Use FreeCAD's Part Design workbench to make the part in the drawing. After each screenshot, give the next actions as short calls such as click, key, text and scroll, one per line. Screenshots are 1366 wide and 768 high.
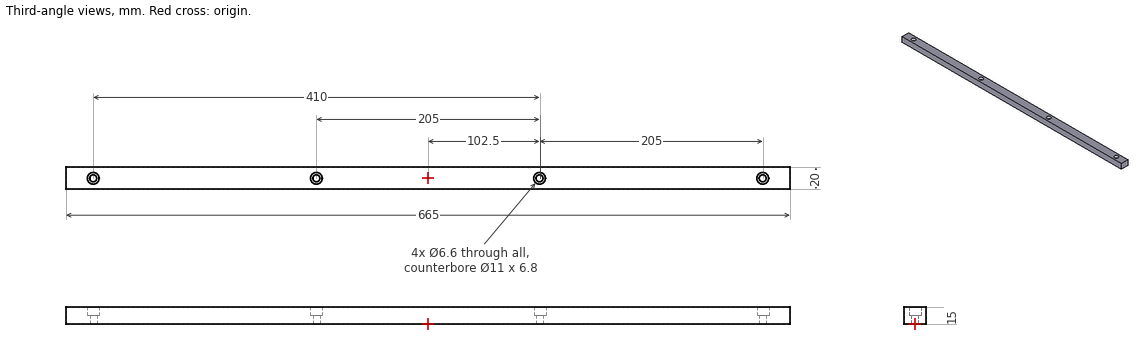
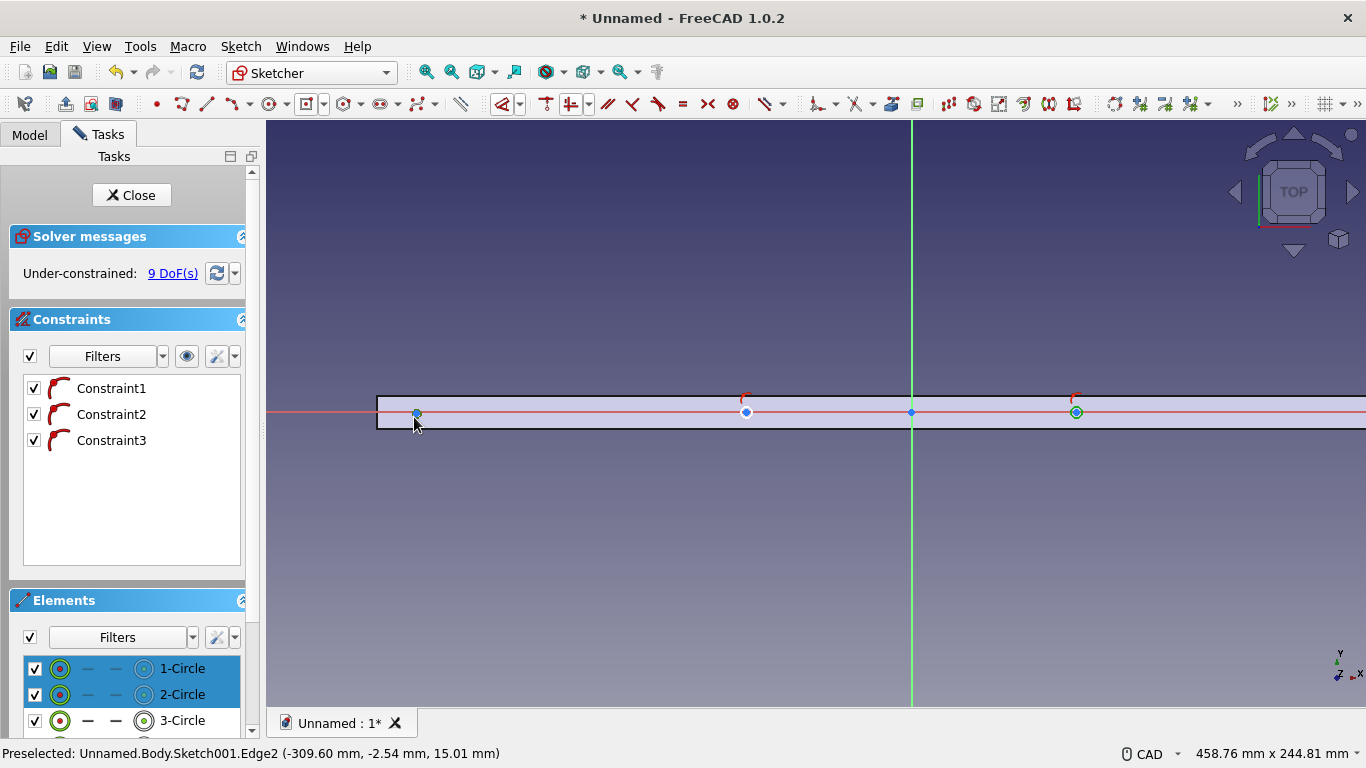
scroll(1082, 411, up, 9)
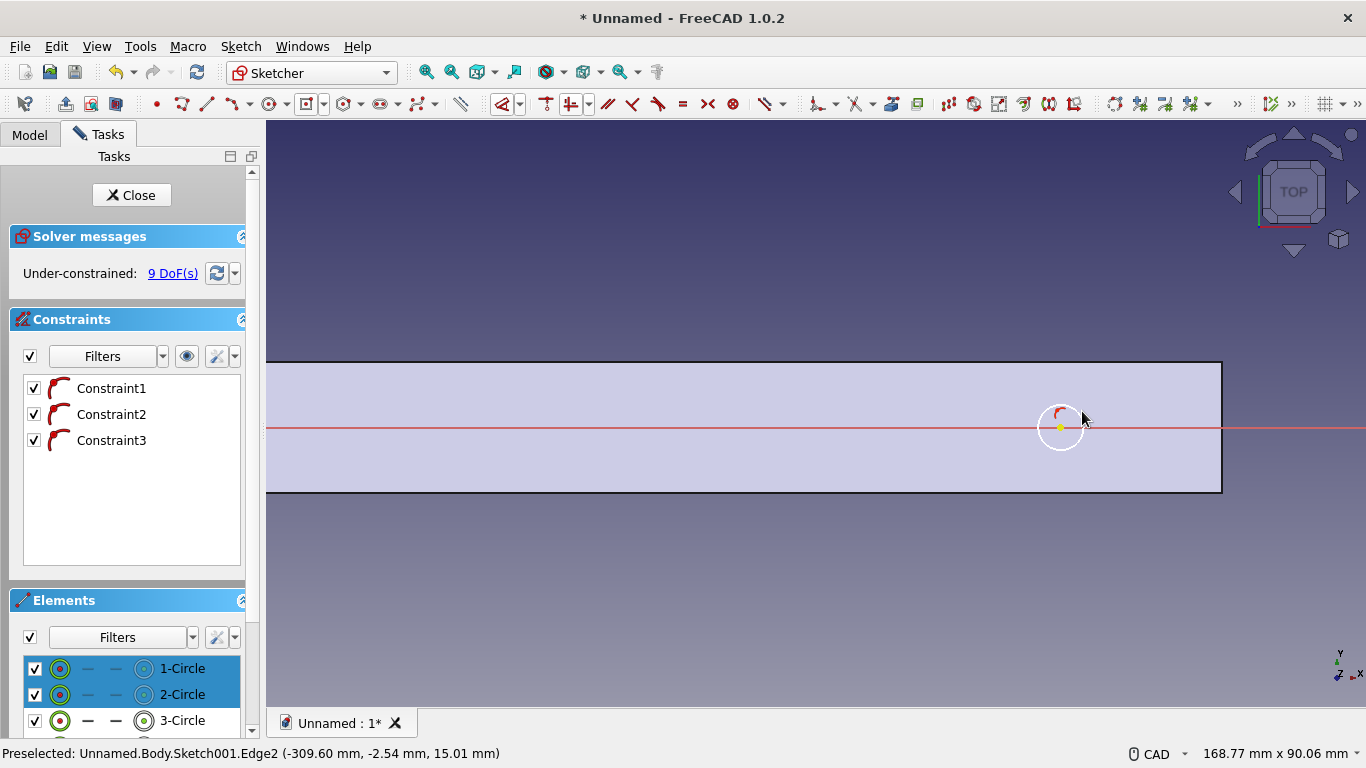
click(1077, 411)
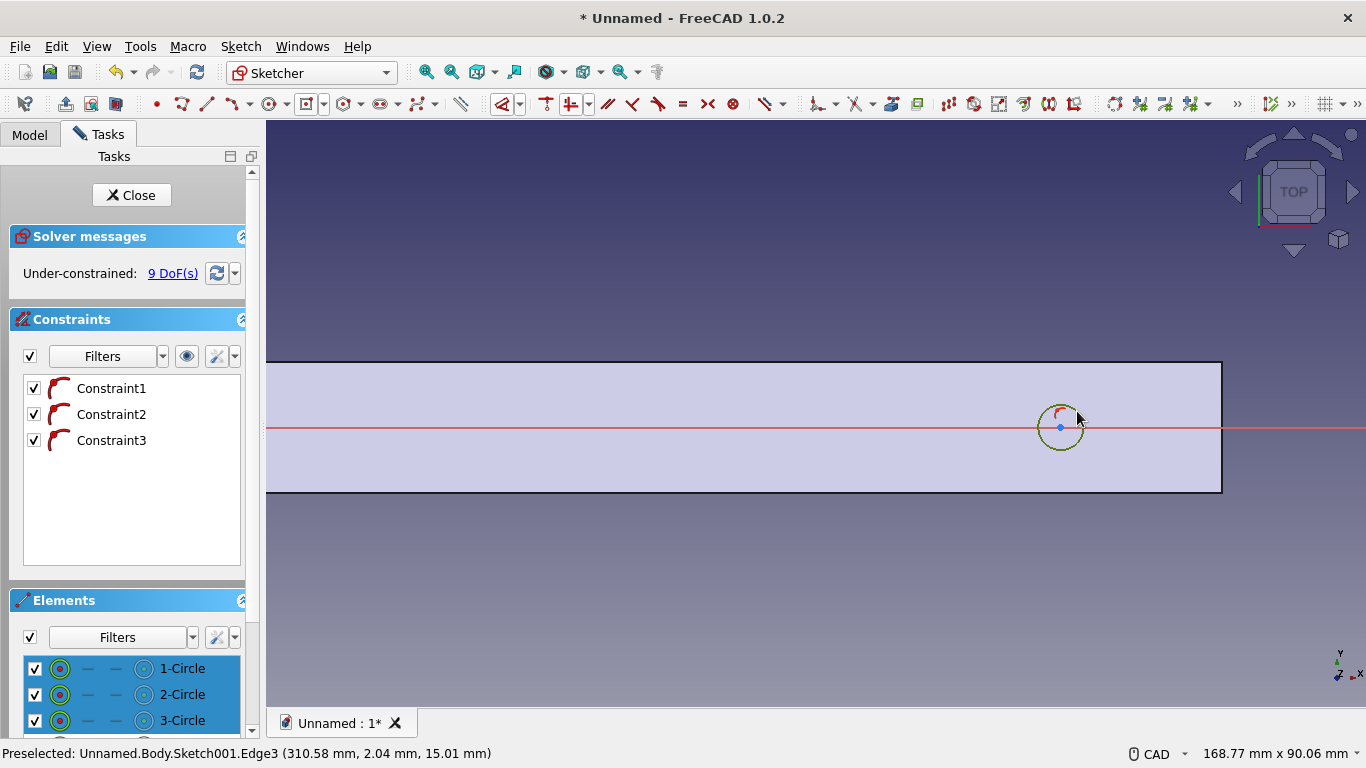
scroll(1083, 411, down, 9)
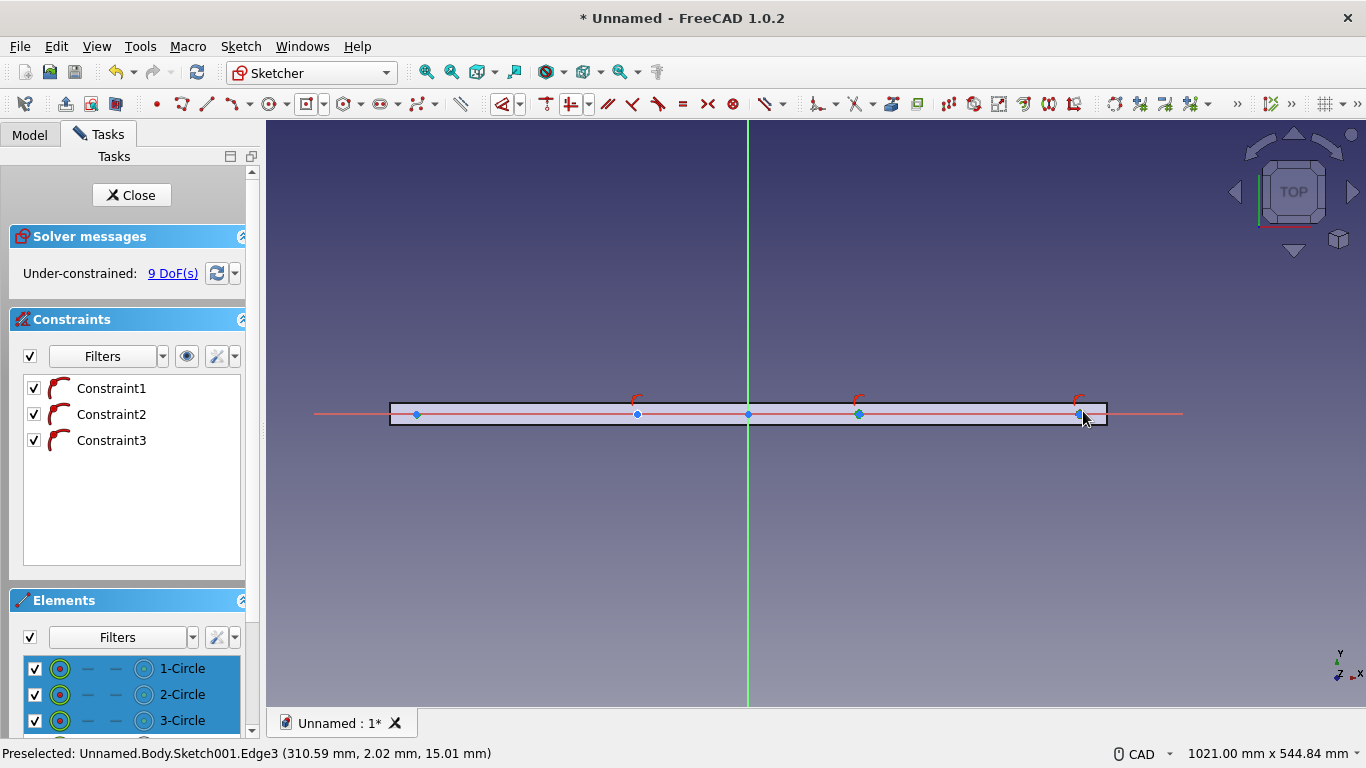
scroll(640, 412, up, 9)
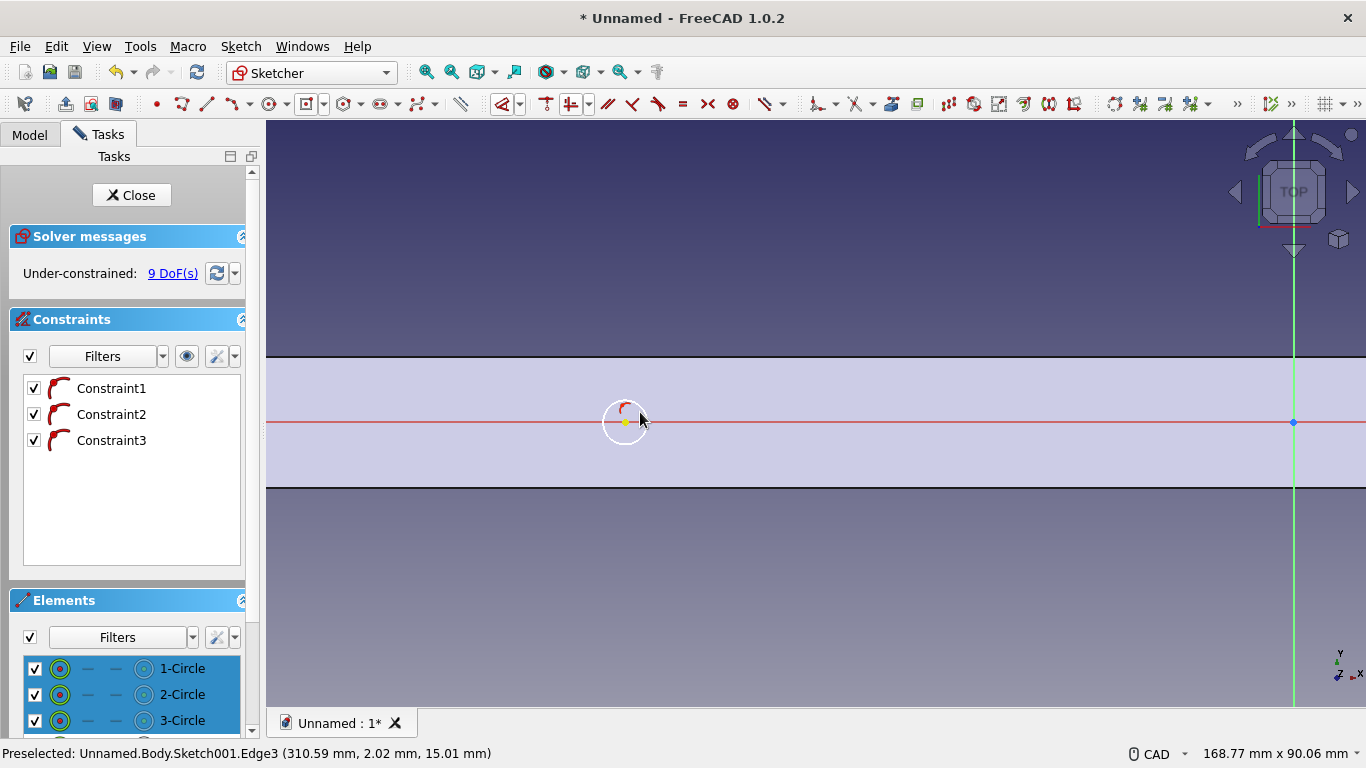
click(641, 407)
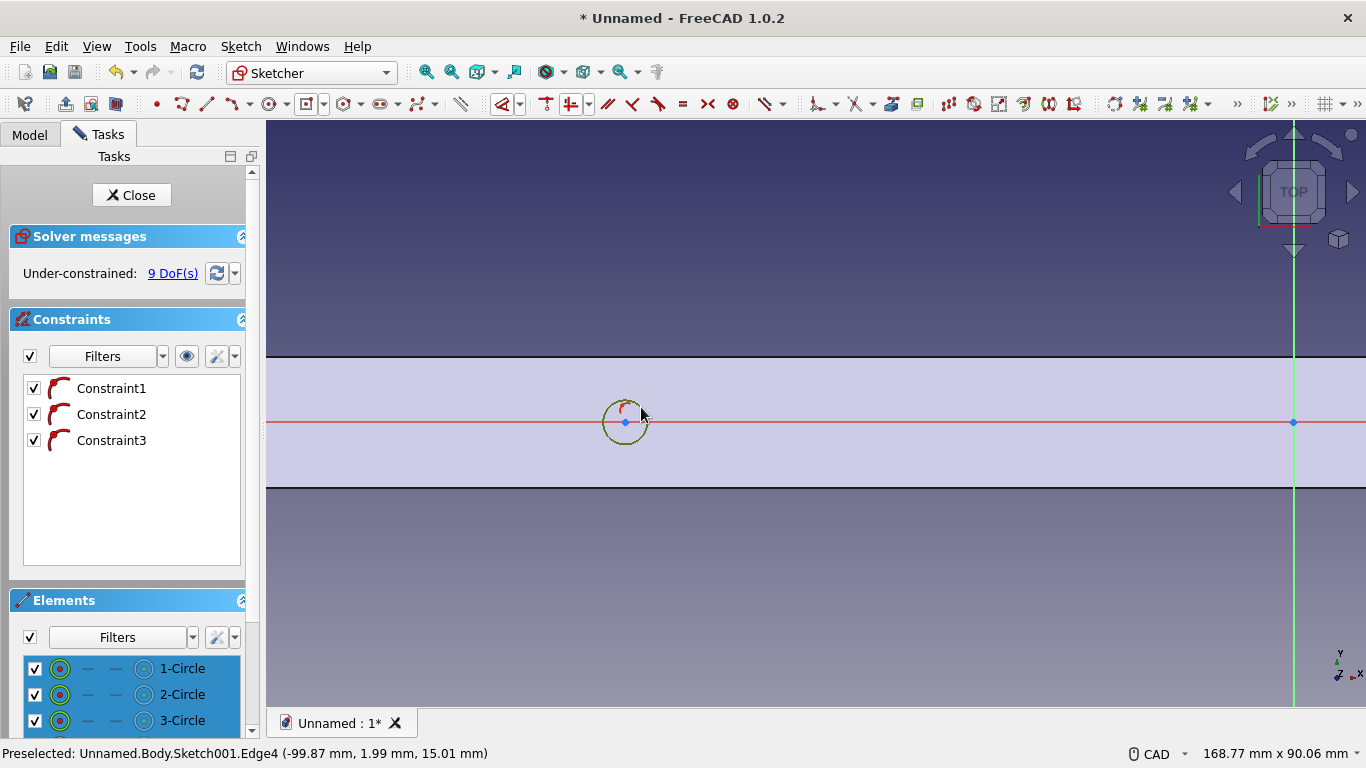
click(683, 104)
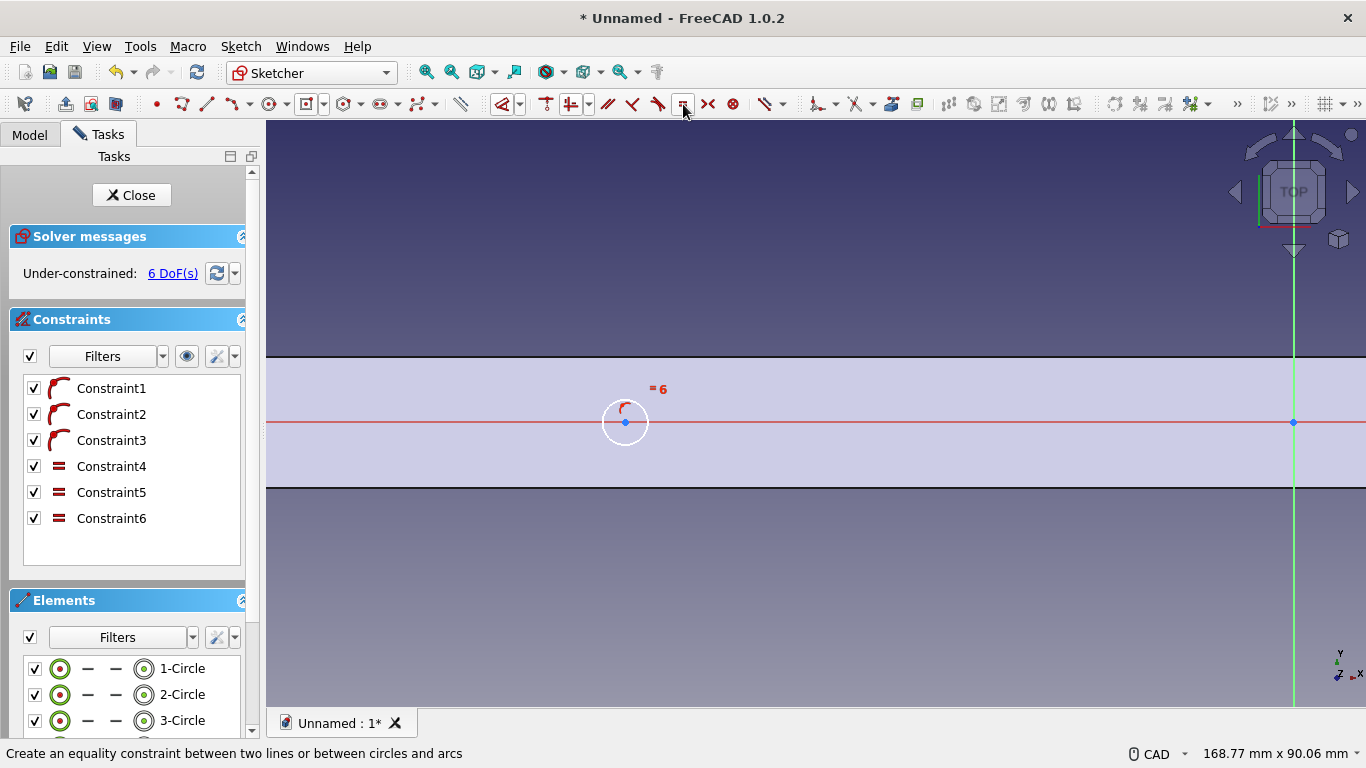
scroll(639, 412, down, 9)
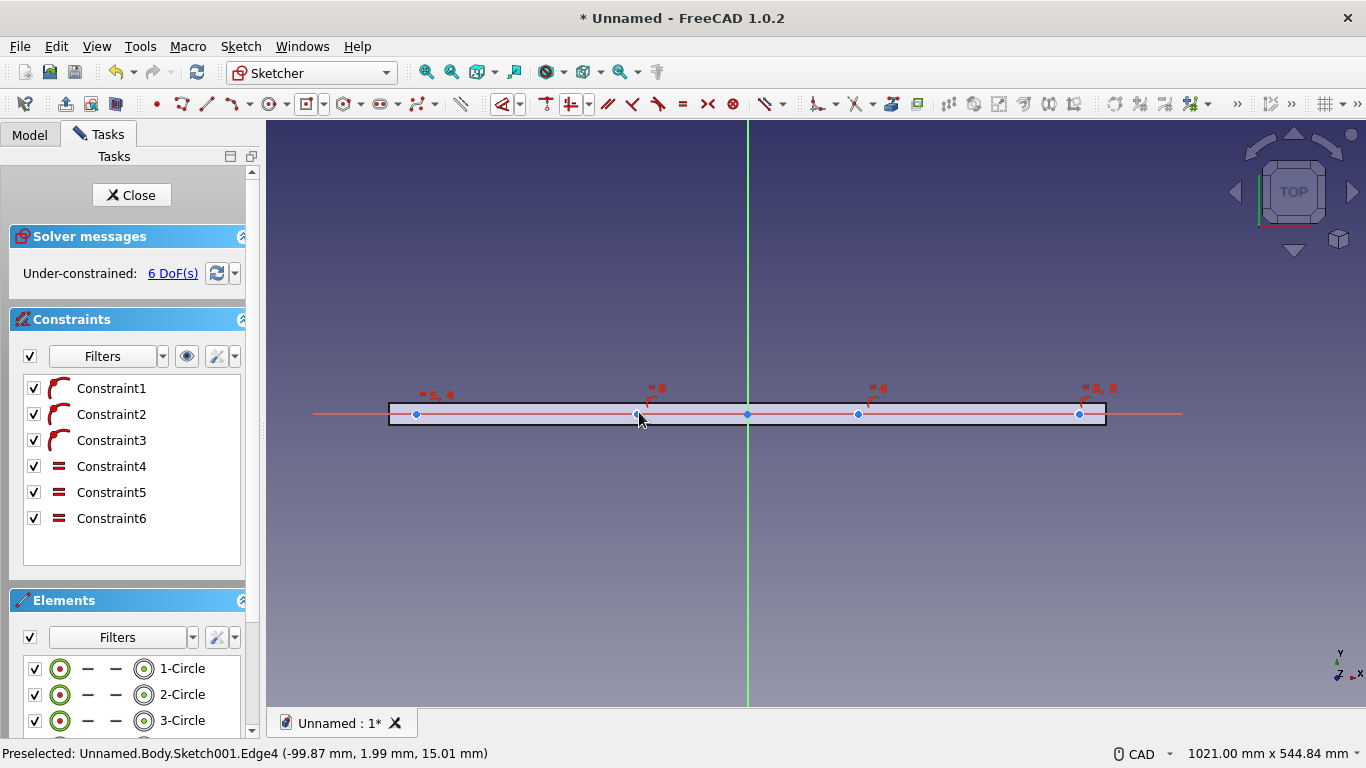
click(416, 415)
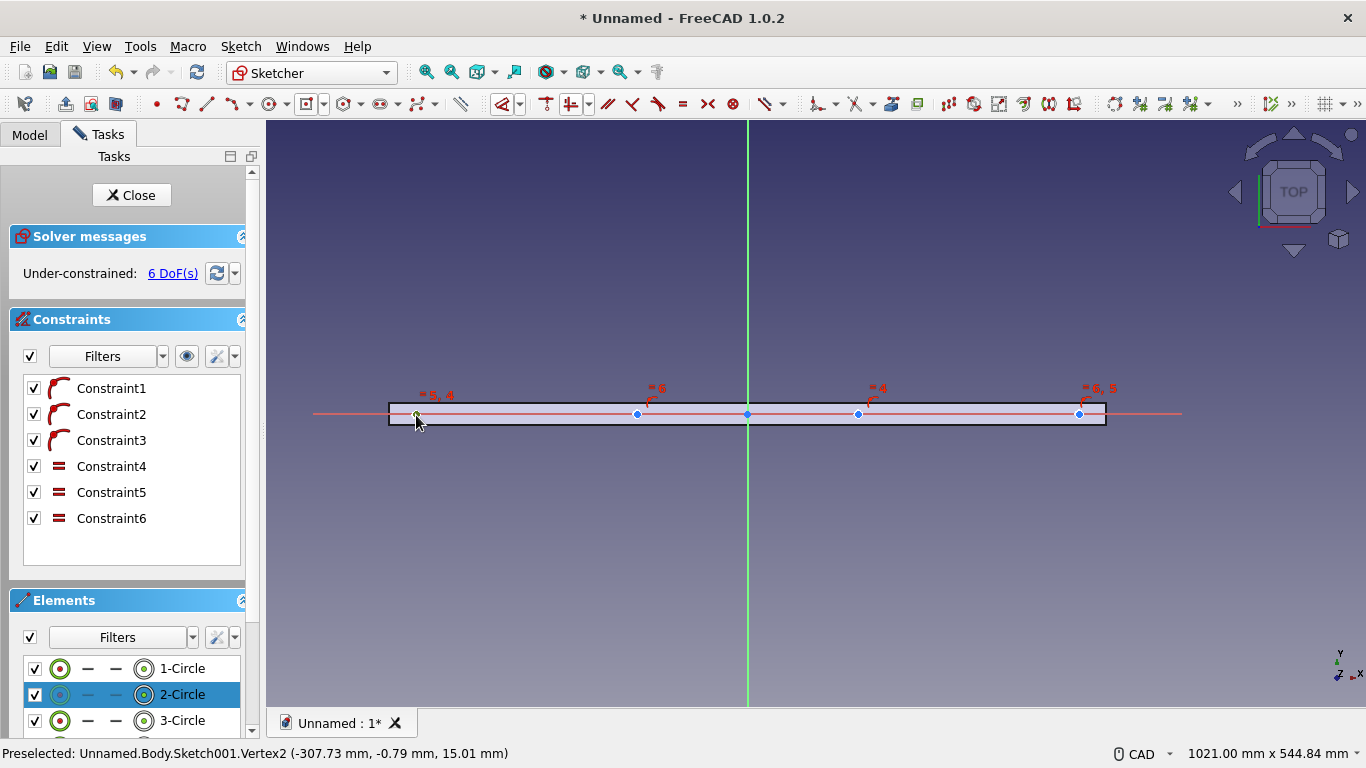
click(359, 414)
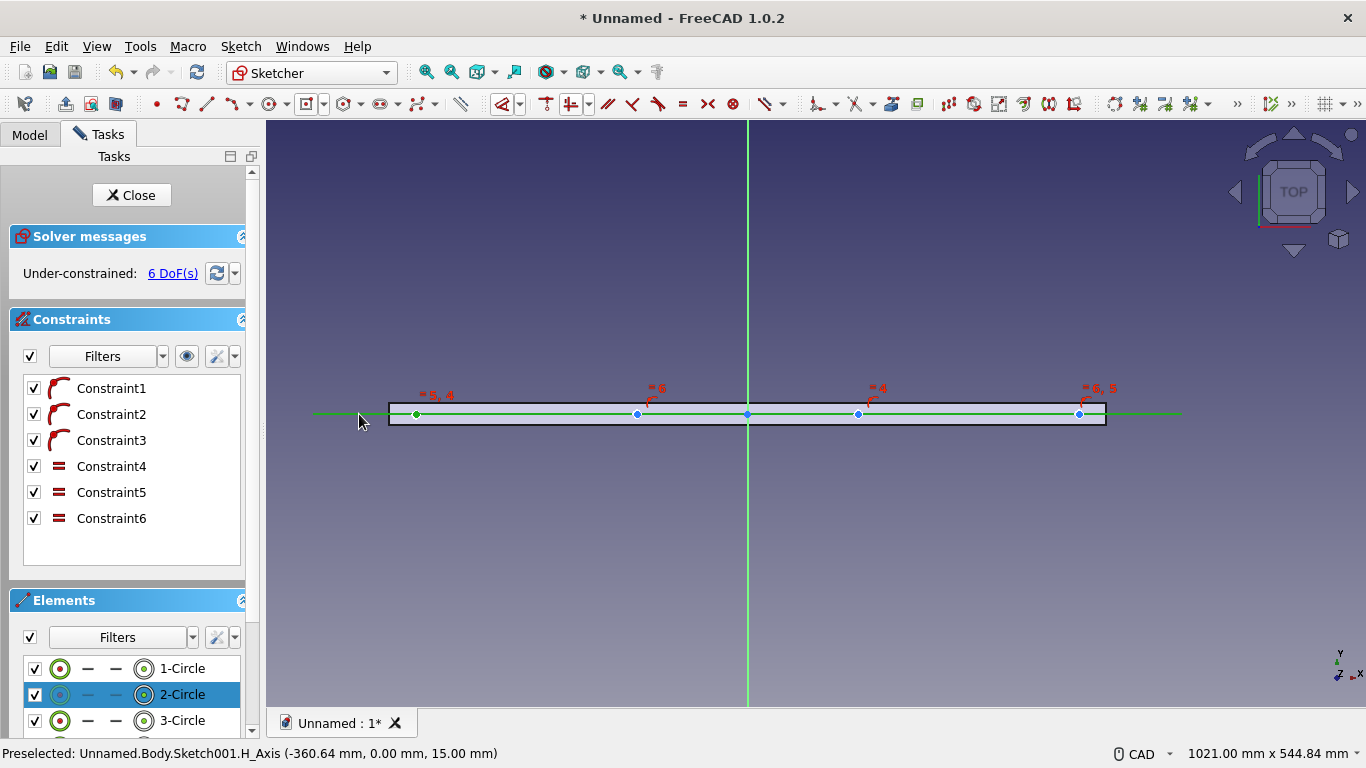
click(546, 104)